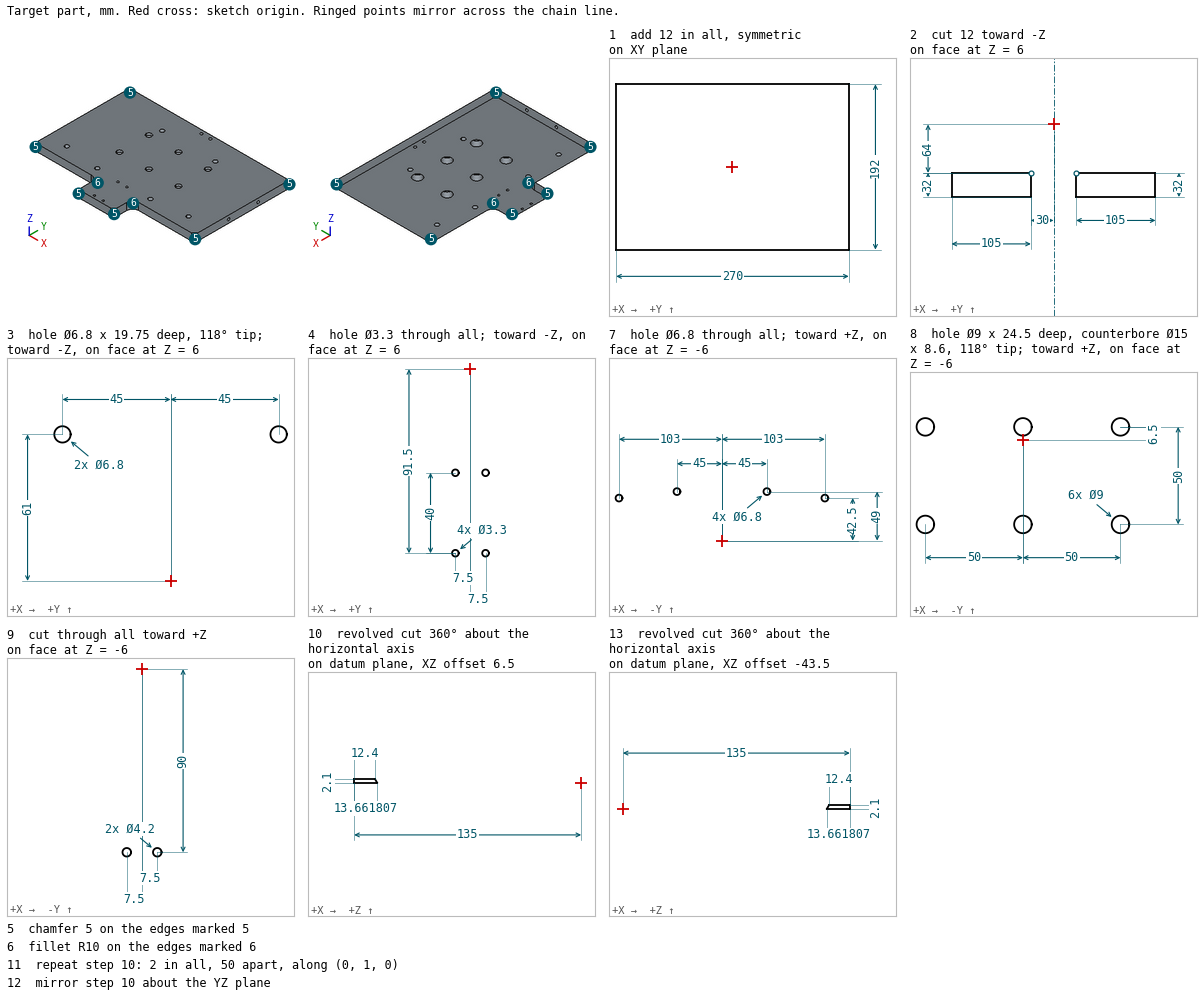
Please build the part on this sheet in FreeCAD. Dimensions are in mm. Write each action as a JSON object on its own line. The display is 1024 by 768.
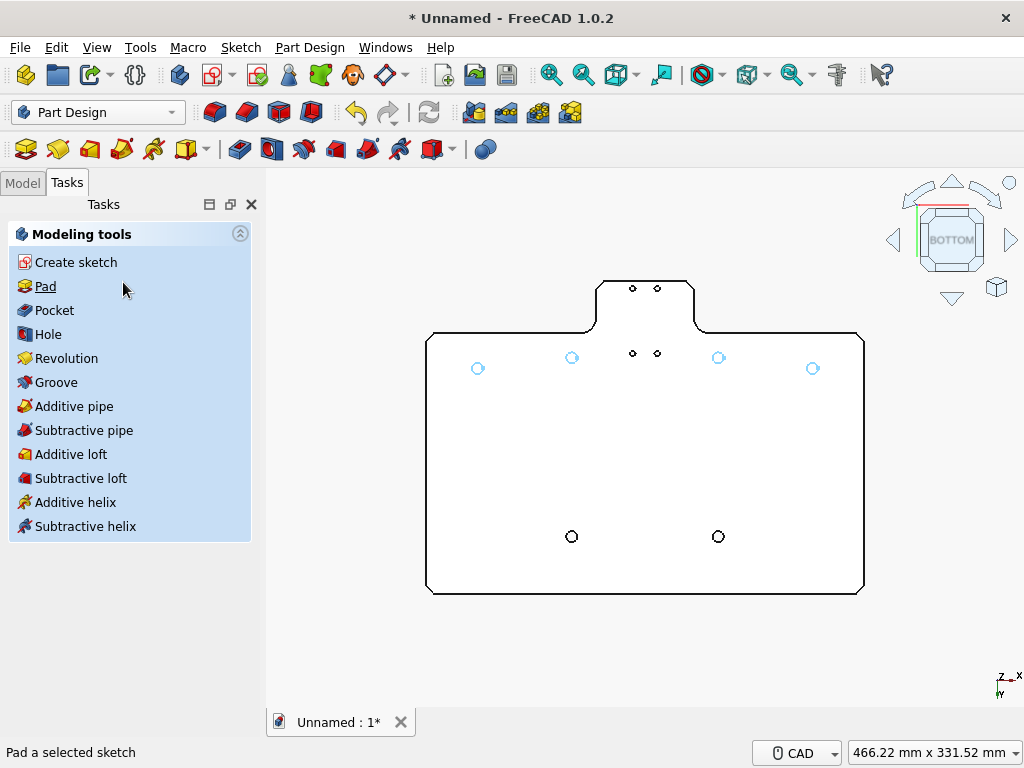
{"action": "left_click", "coordinate": [272, 150]}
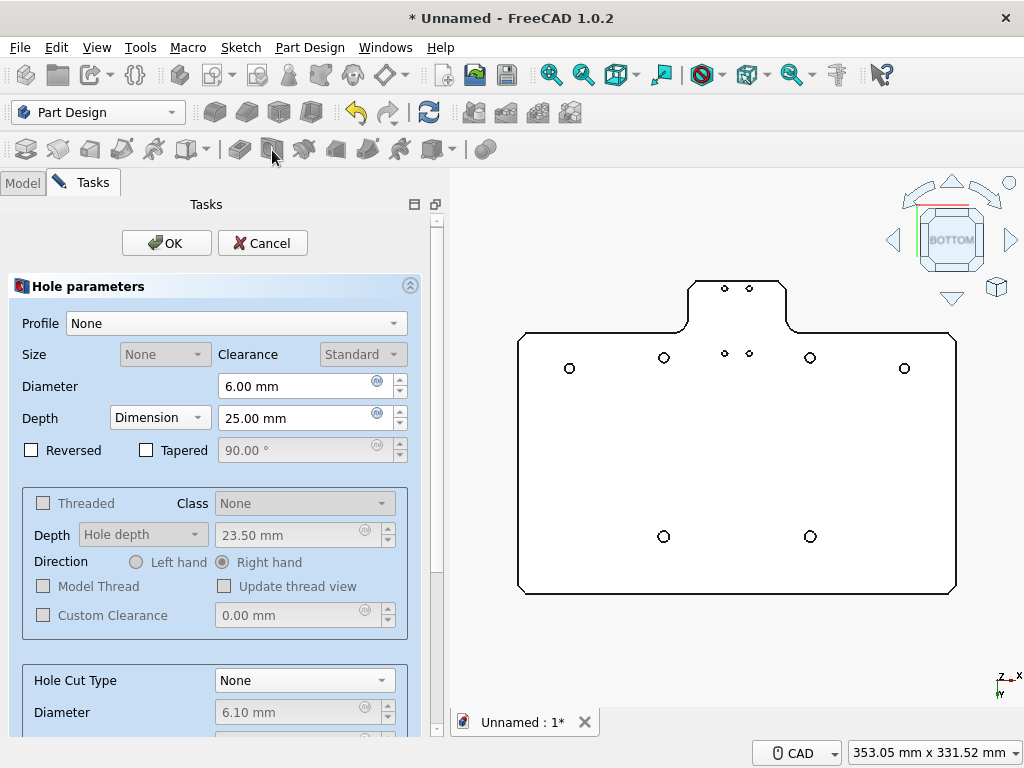
{"action": "triple_click", "coordinate": [305, 386]}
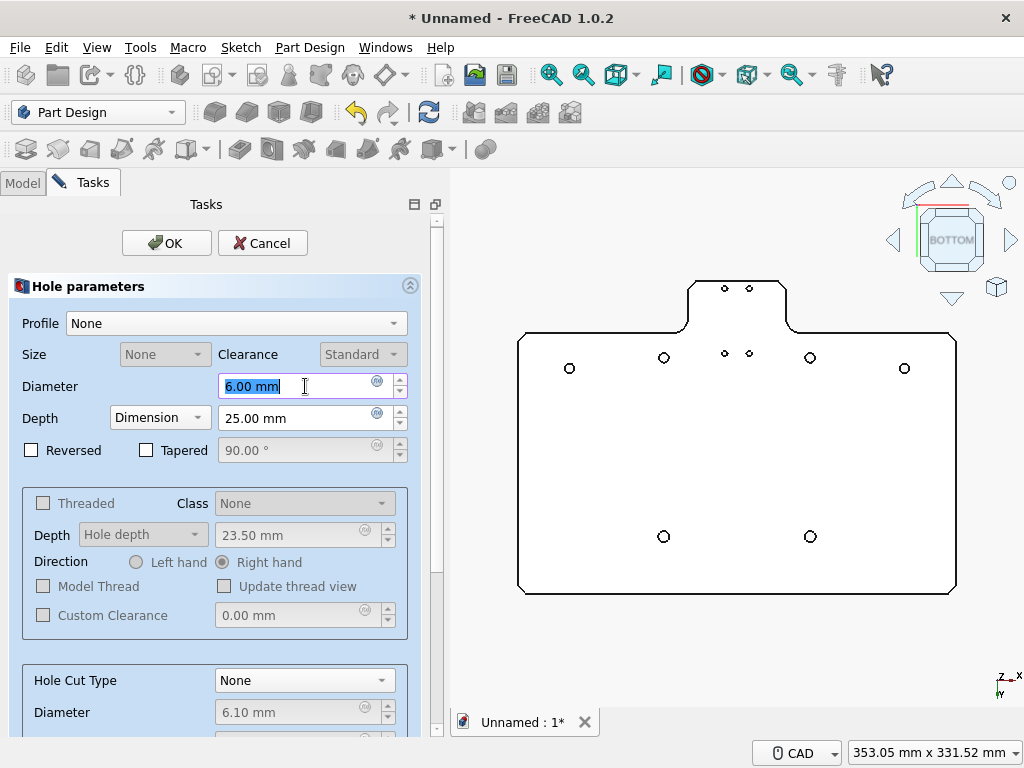
{"action": "type", "text": "6.8"}
{"action": "key", "text": "Tab"}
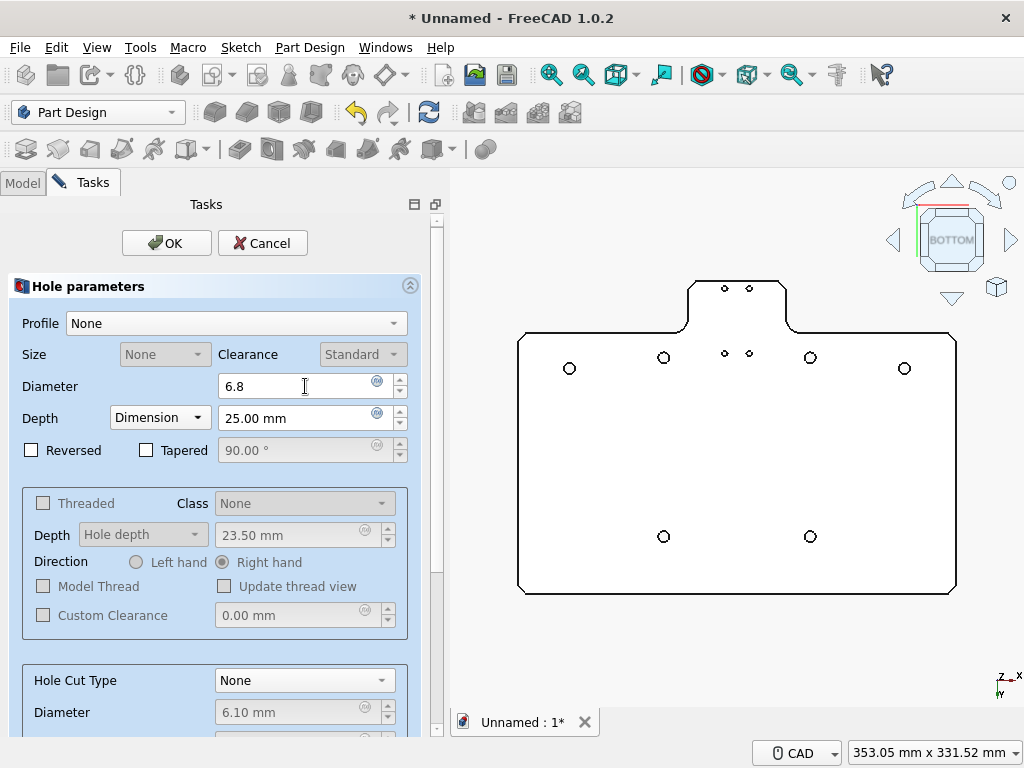
{"action": "left_click", "coordinate": [161, 418]}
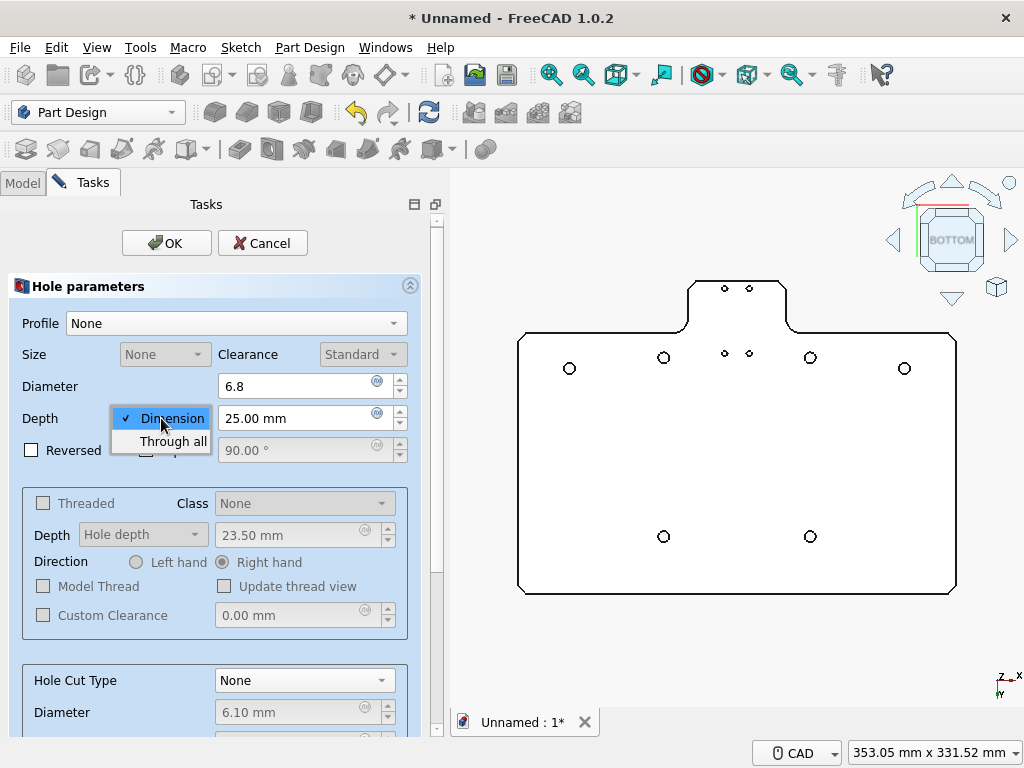
{"action": "left_click", "coordinate": [160, 442]}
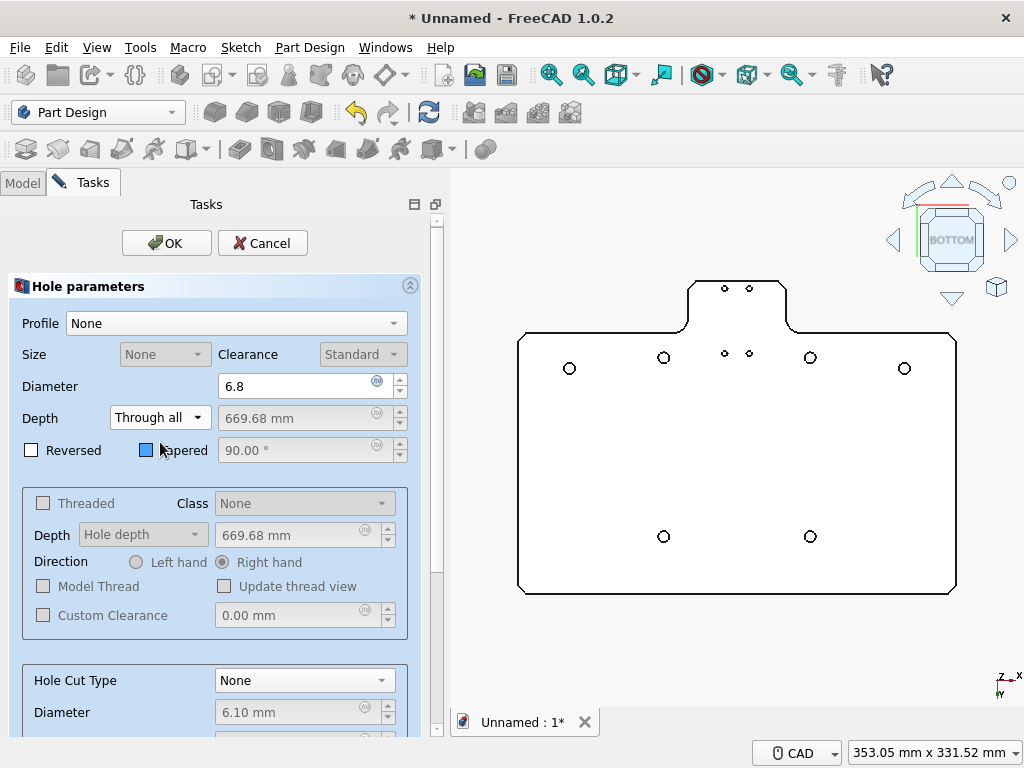
{"action": "left_click", "coordinate": [167, 243]}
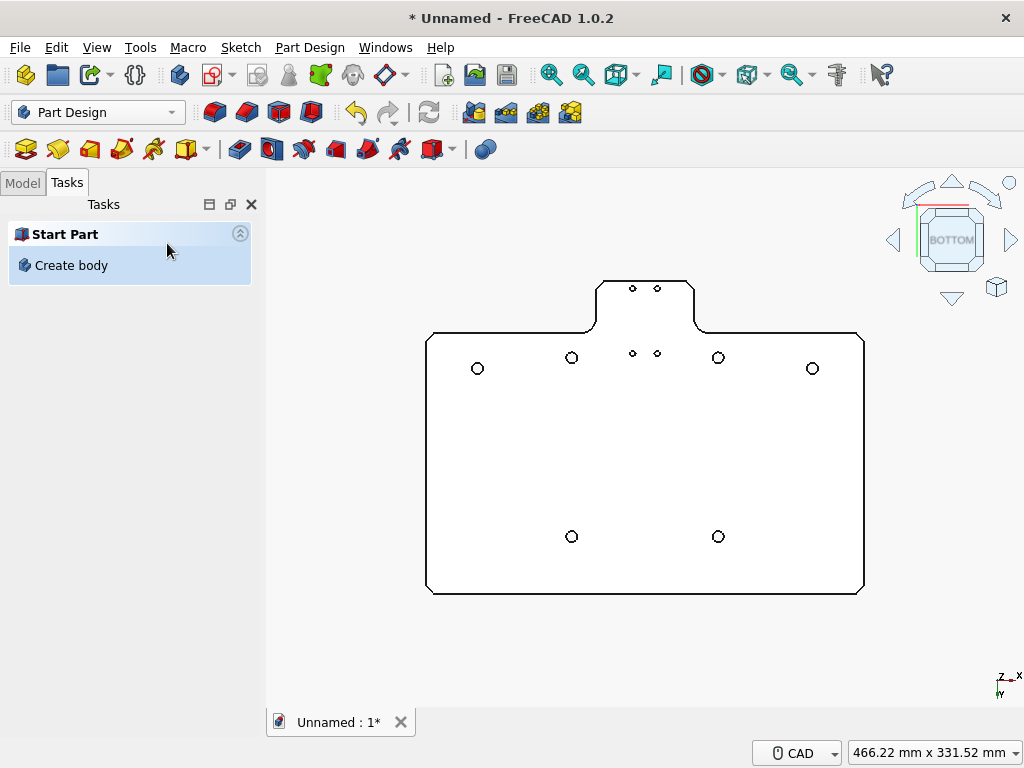
{"action": "left_click", "coordinate": [645, 481]}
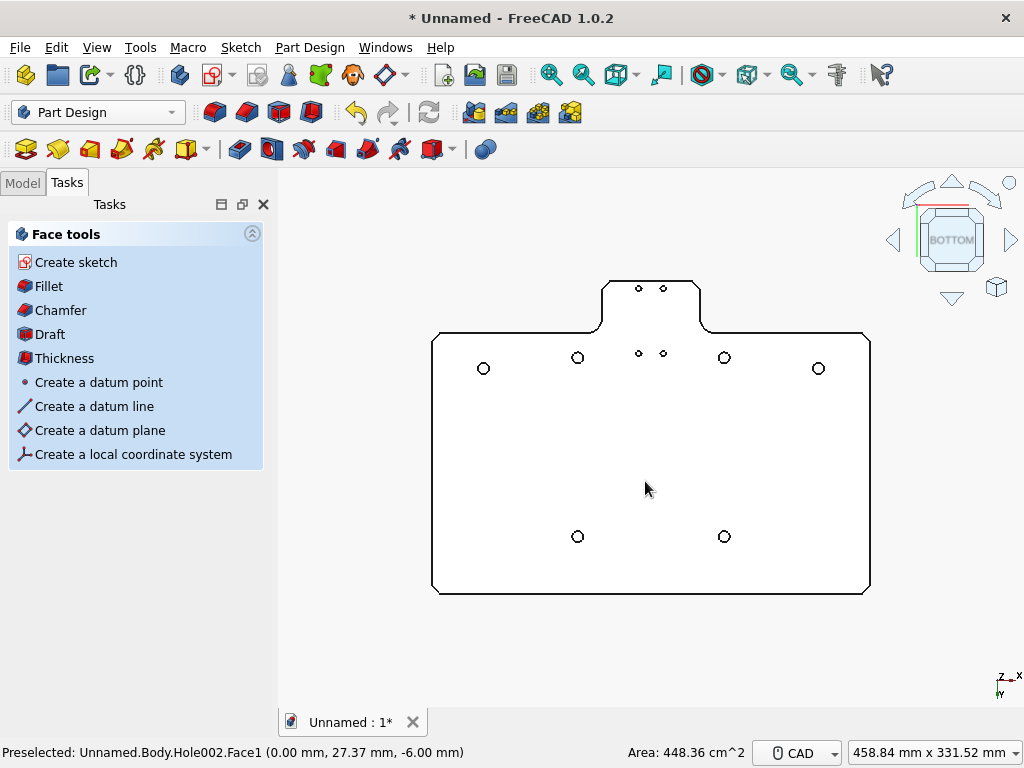
{"action": "left_click", "coordinate": [212, 76]}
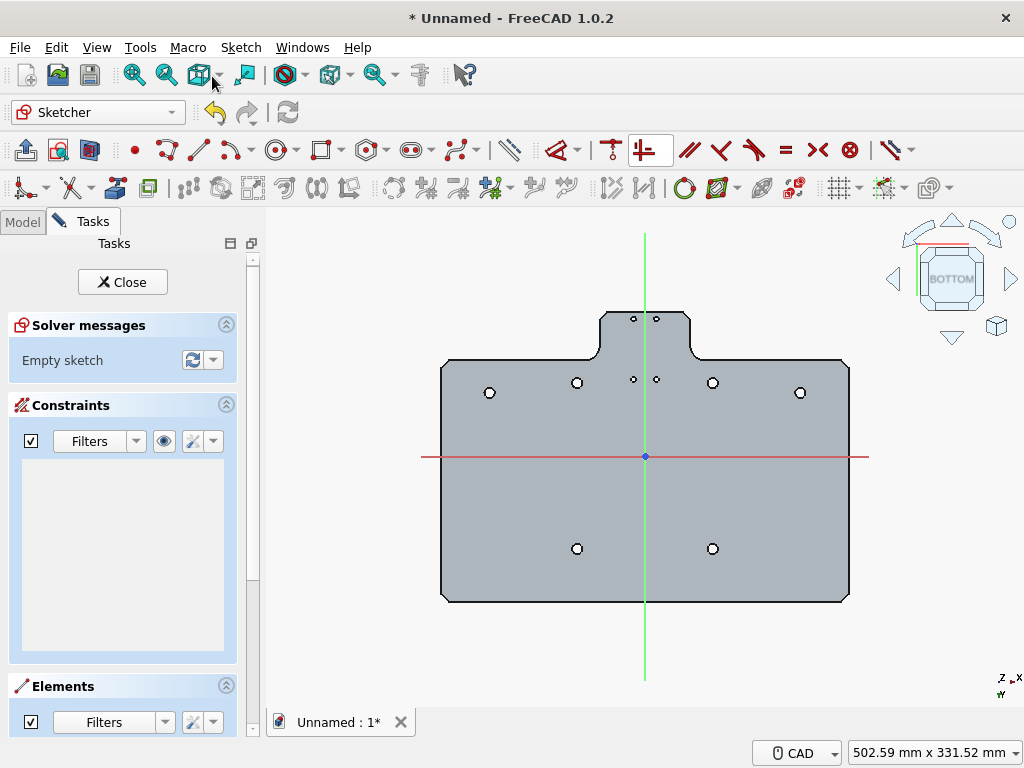
{"action": "scroll", "coordinate": [701, 508], "scroll_direction": "up", "scroll_amount": 4}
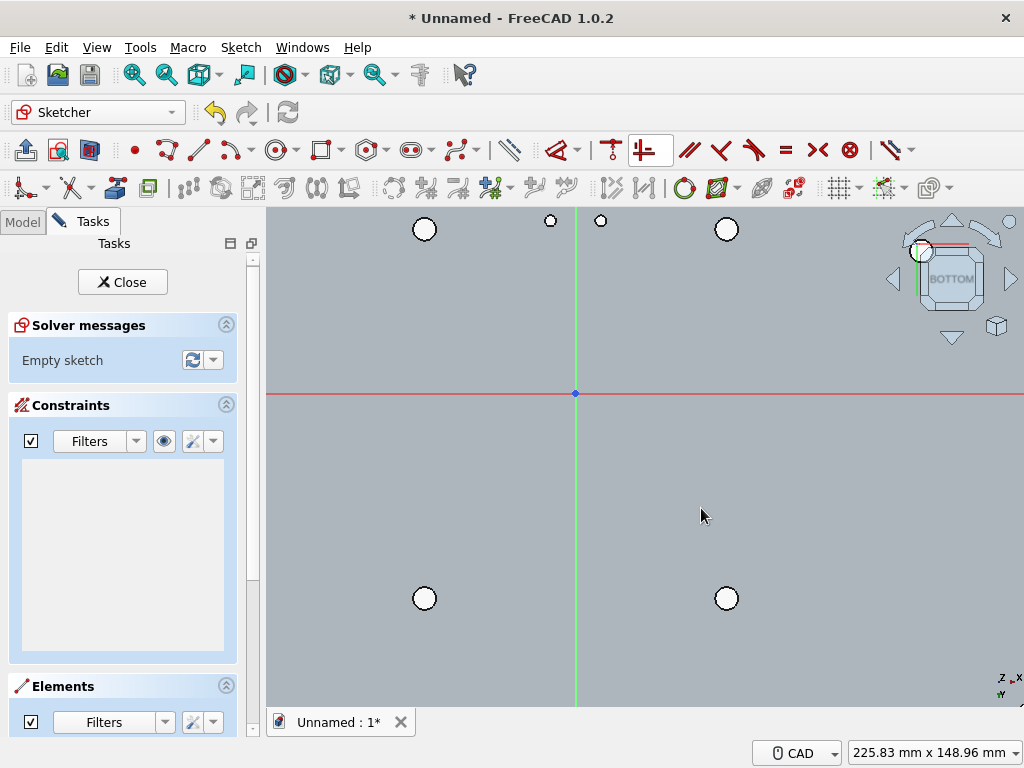
{"action": "left_click", "coordinate": [276, 150]}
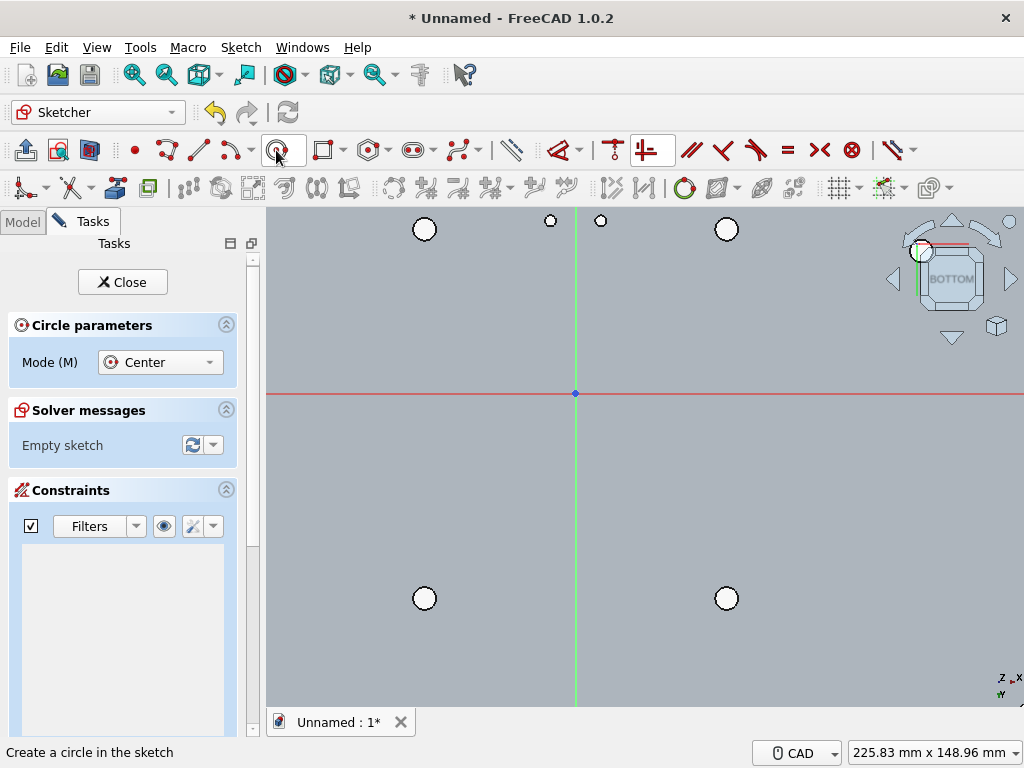
{"action": "scroll", "coordinate": [743, 540], "scroll_direction": "up", "scroll_amount": 3}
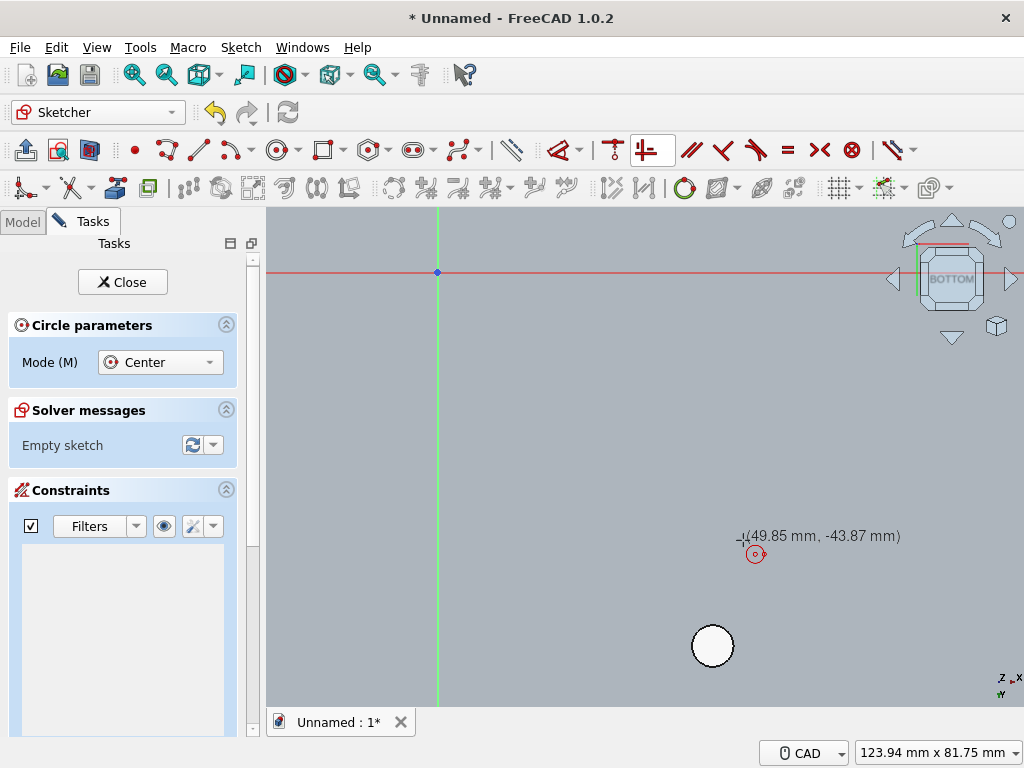
{"action": "left_click", "coordinate": [743, 539]}
{"action": "mouse_move", "coordinate": [763, 520]}